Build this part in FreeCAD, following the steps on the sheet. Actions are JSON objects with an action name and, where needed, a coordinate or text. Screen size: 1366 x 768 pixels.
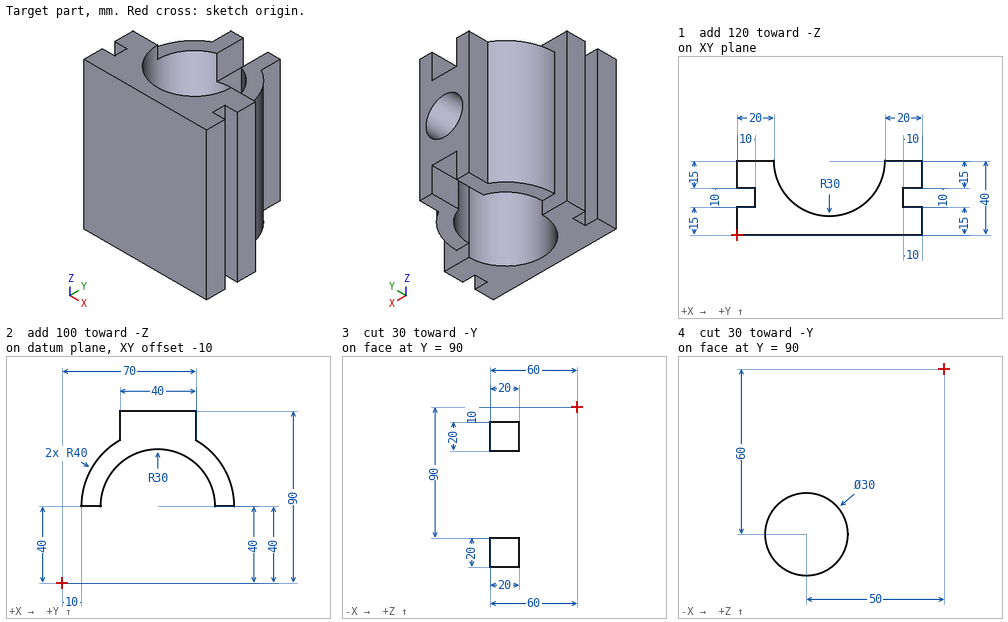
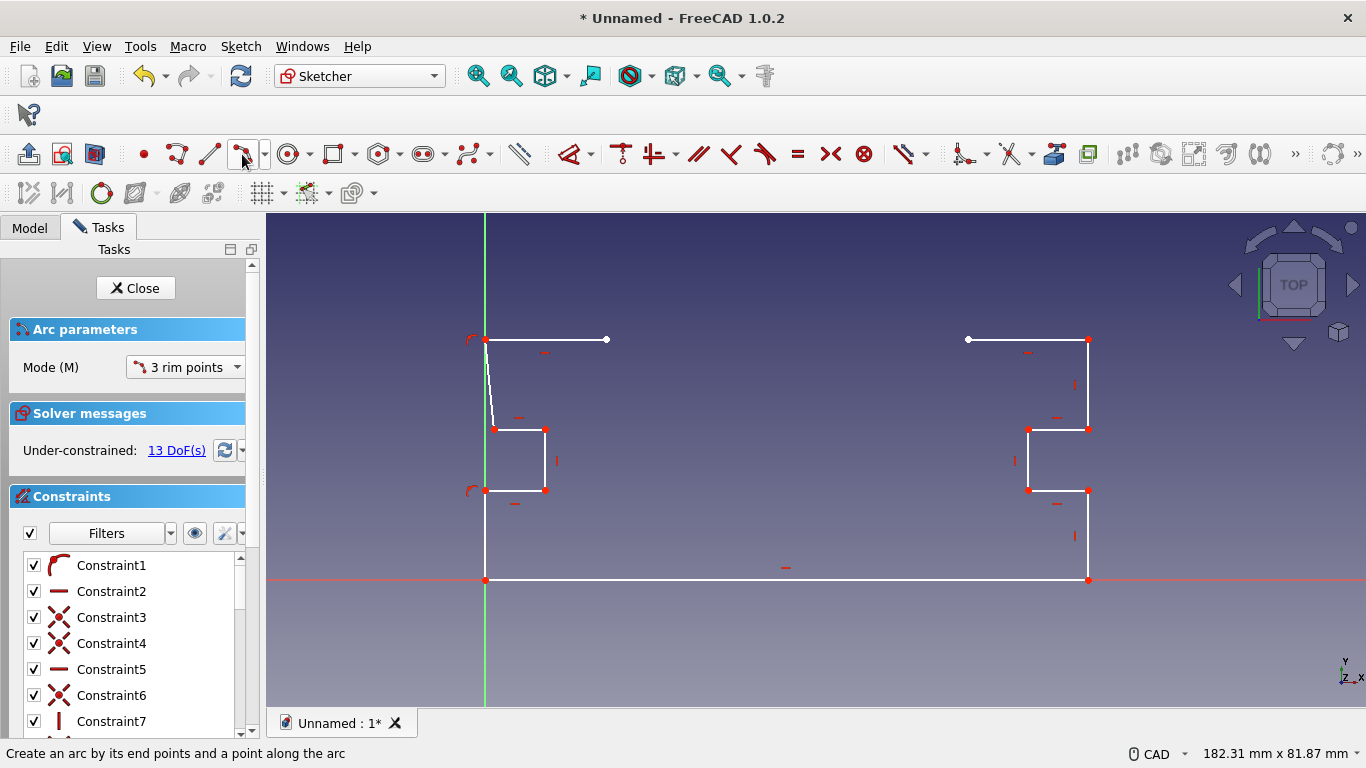
{"action": "left_click", "coordinate": [968, 340]}
{"action": "left_click", "coordinate": [606, 340]}
{"action": "left_click", "coordinate": [787, 520]}
{"action": "key", "text": "Escape"}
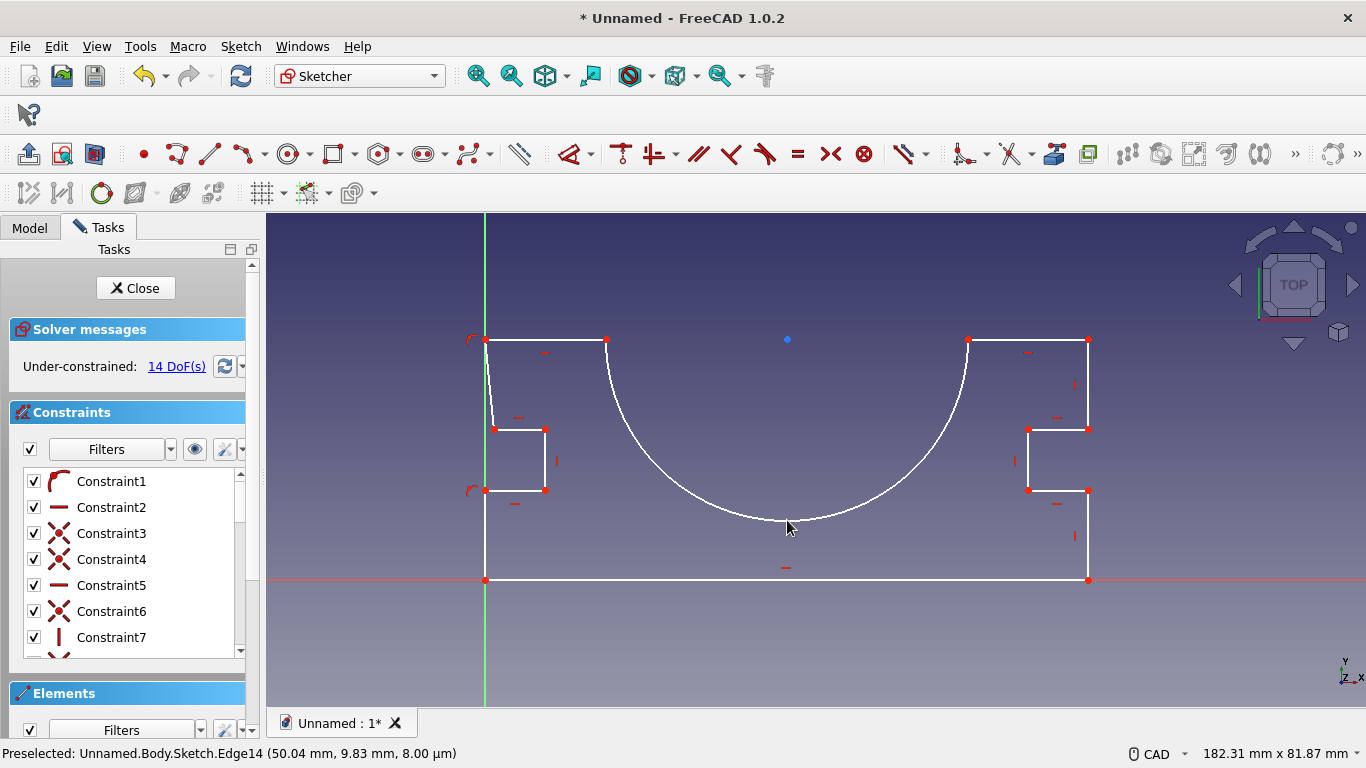
{"action": "left_click", "coordinate": [488, 367]}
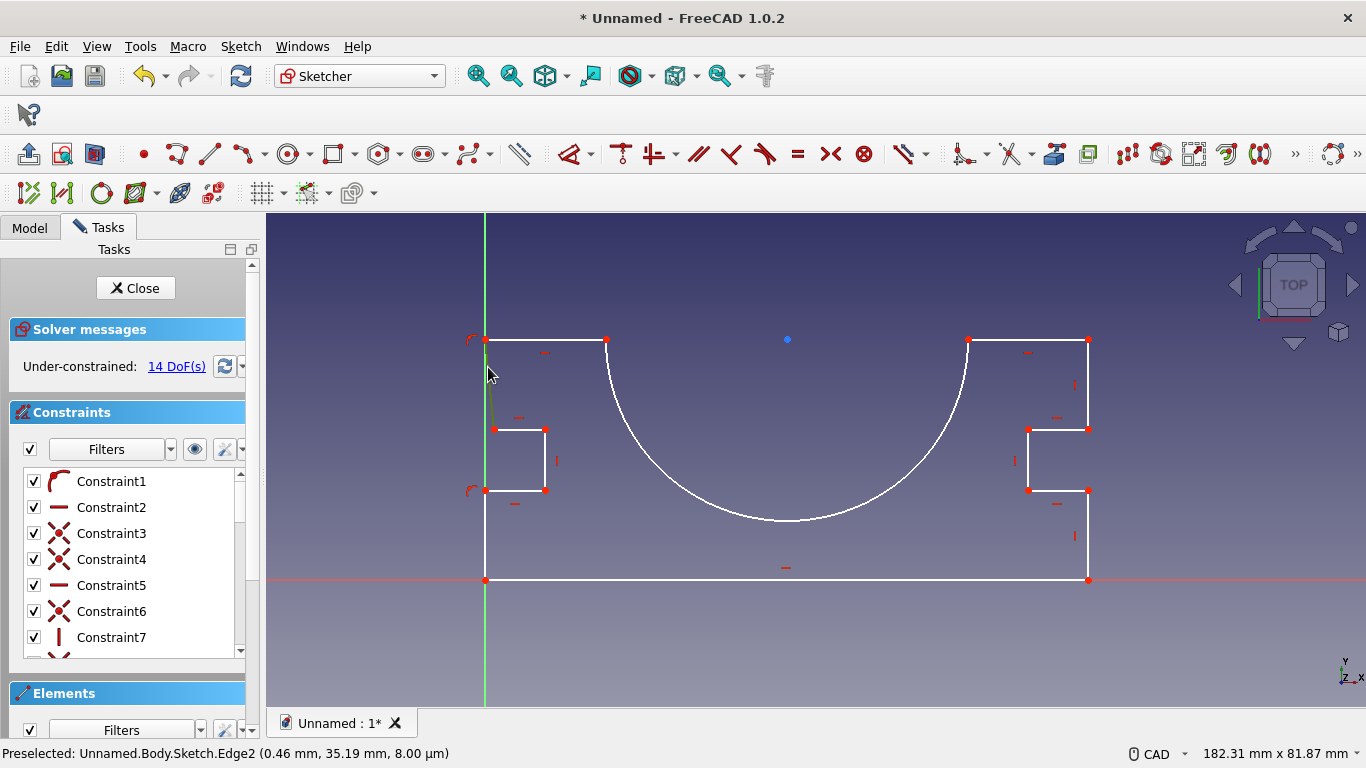
{"action": "left_click", "coordinate": [676, 154]}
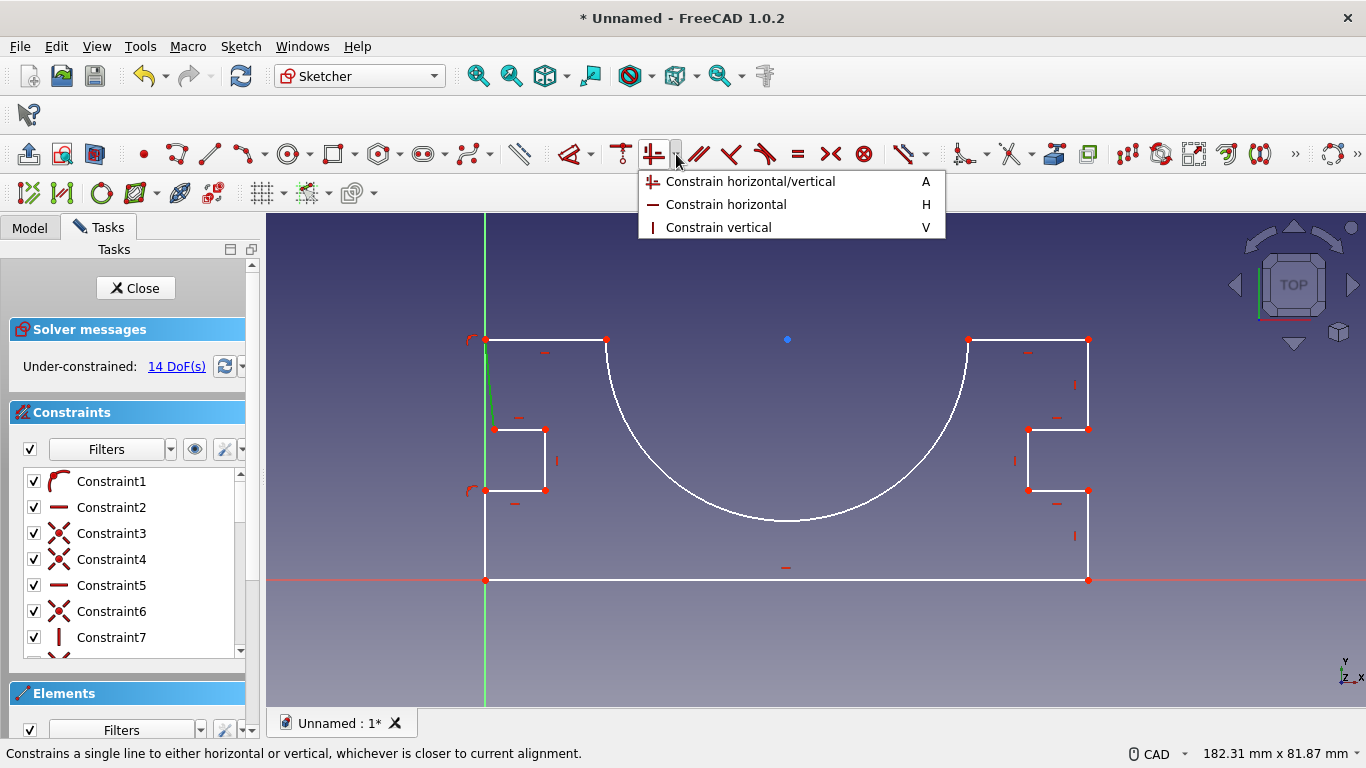
{"action": "left_click", "coordinate": [792, 228]}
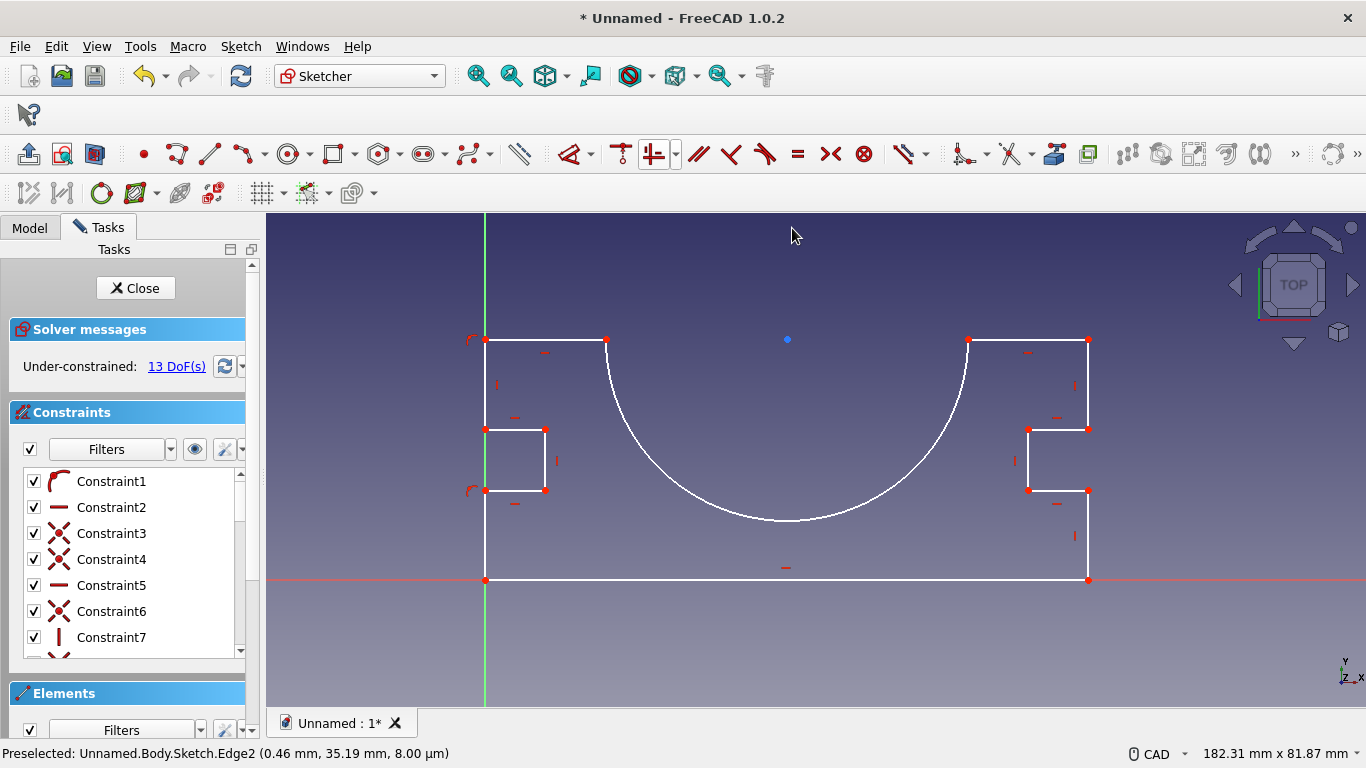
{"action": "left_click", "coordinate": [568, 154]}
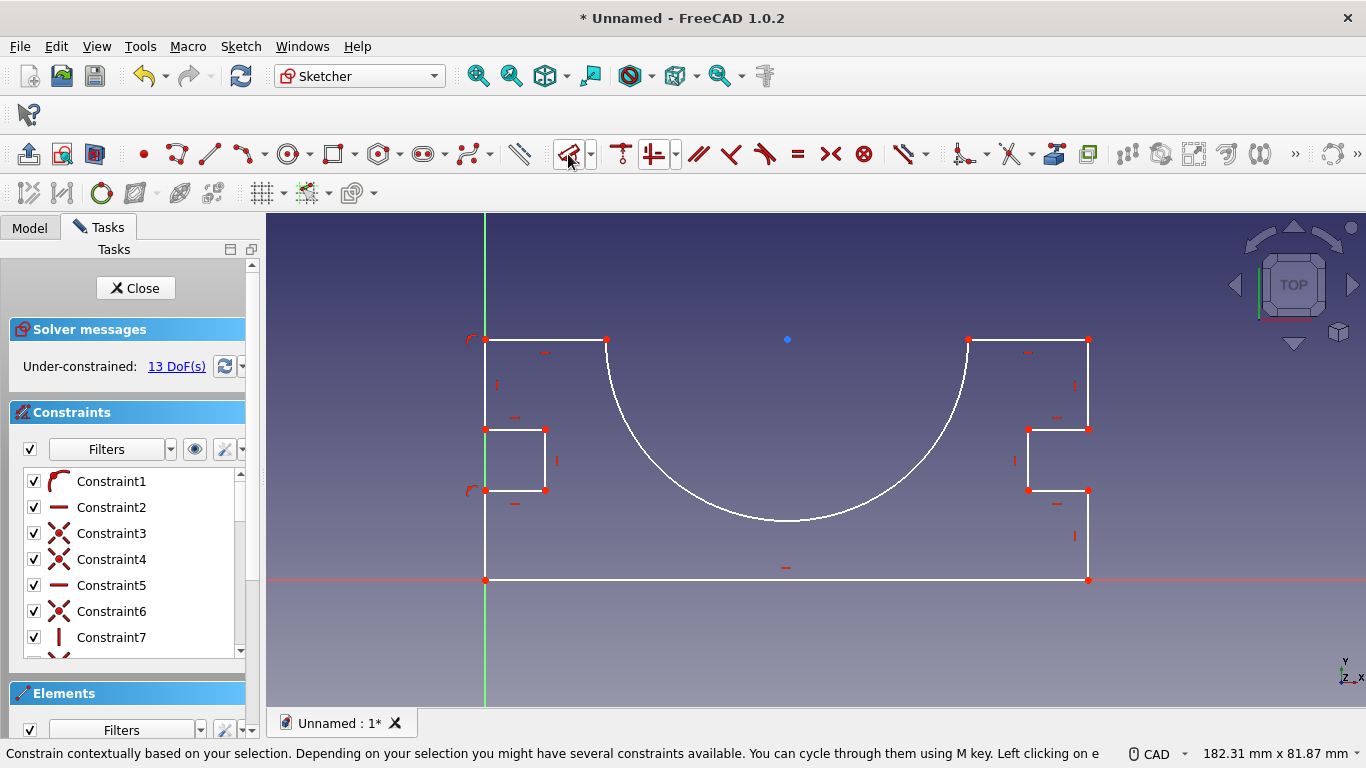
{"action": "left_click", "coordinate": [681, 486]}
{"action": "left_click", "coordinate": [662, 512]}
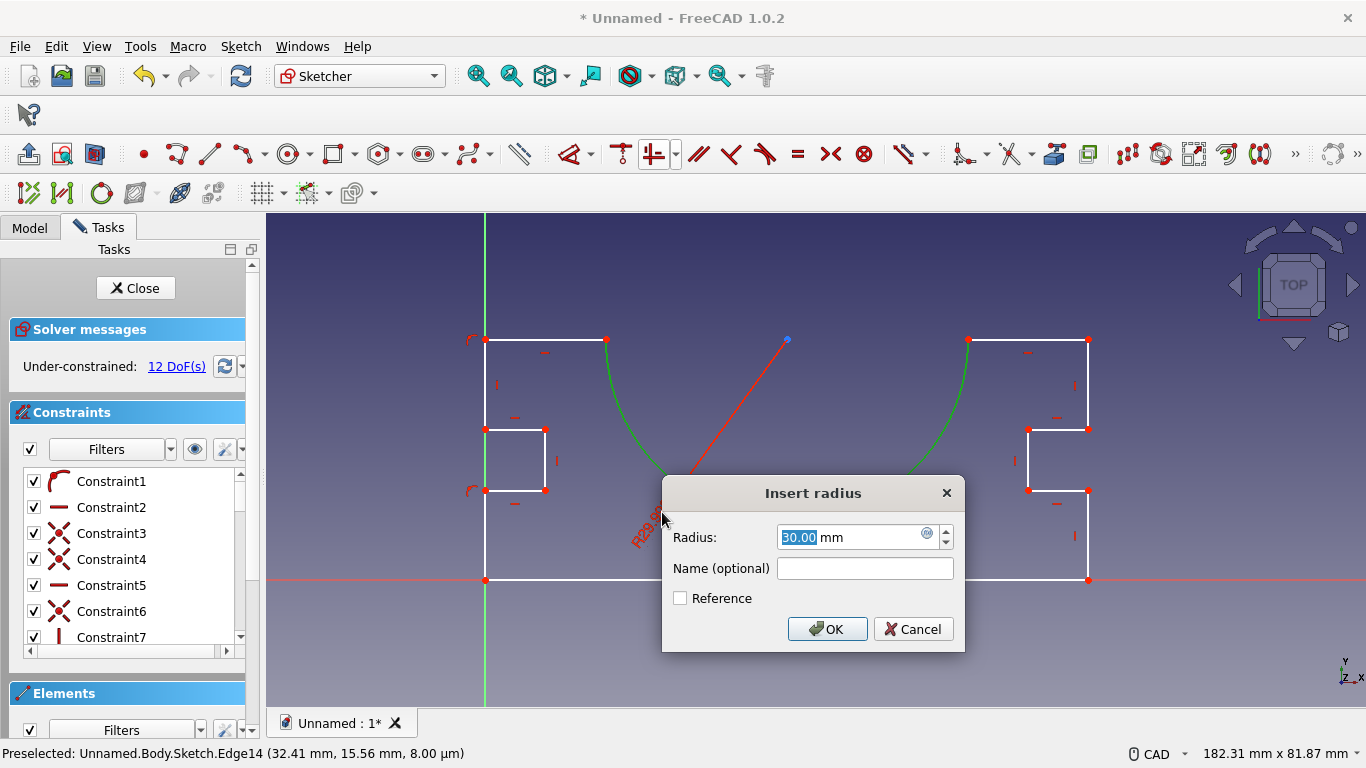
{"action": "type", "text": "30"}
{"action": "key", "text": "Return"}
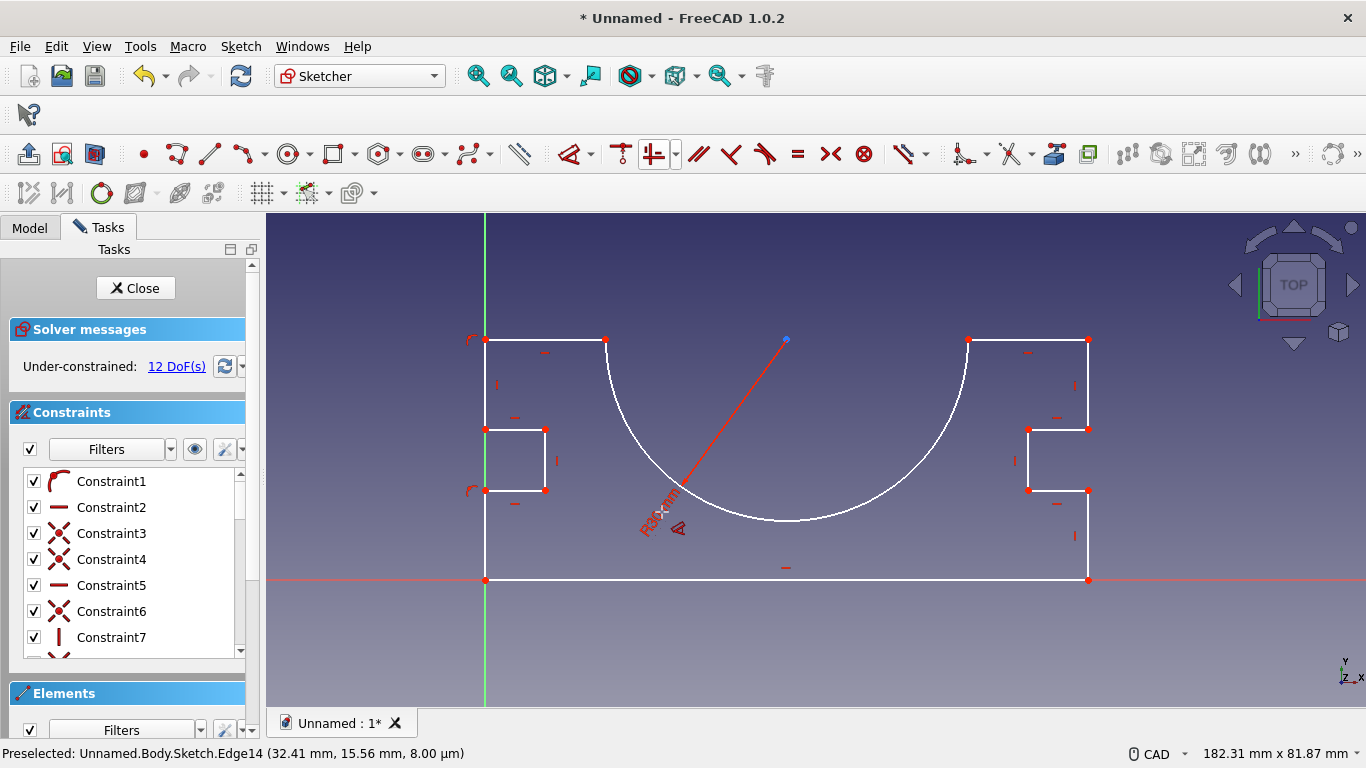
{"action": "left_click", "coordinate": [570, 340]}
{"action": "left_click", "coordinate": [546, 306]}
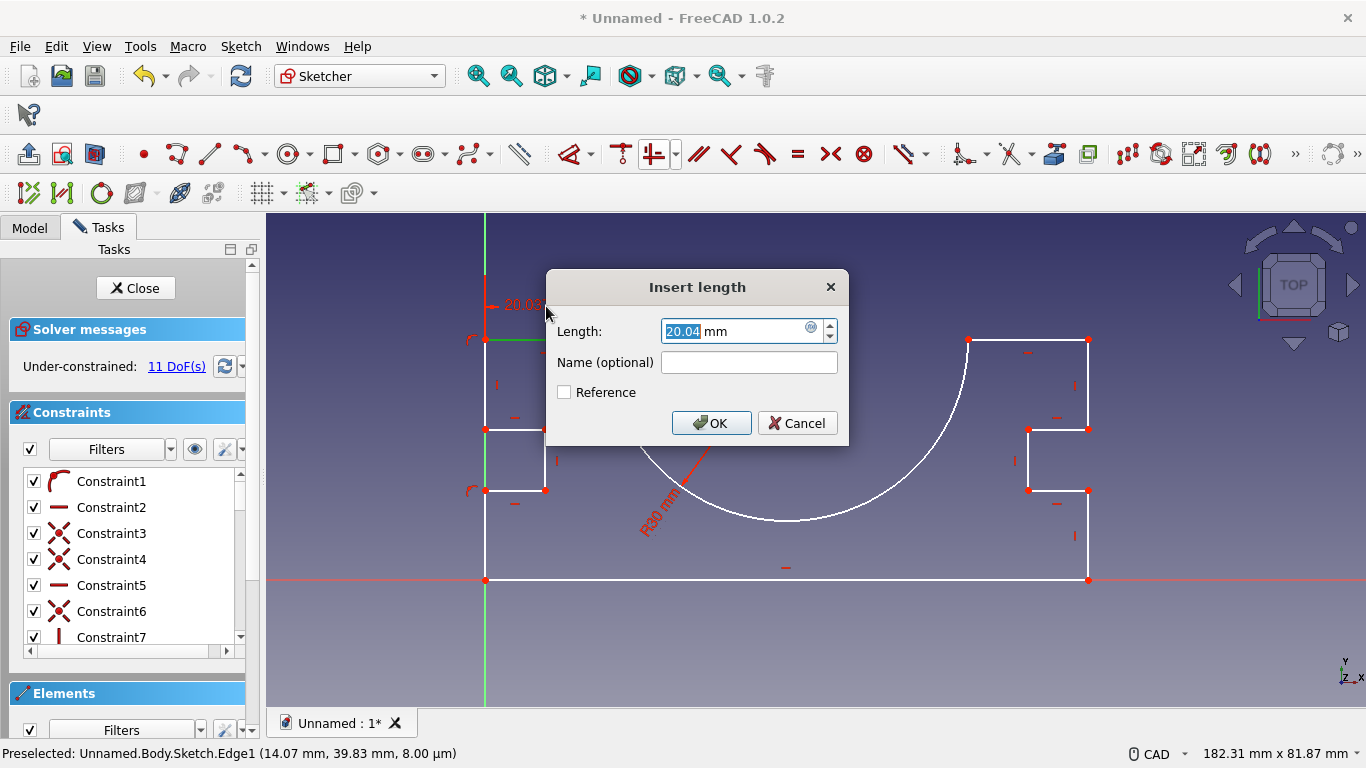
{"action": "type", "text": "20"}
{"action": "key", "text": "Return"}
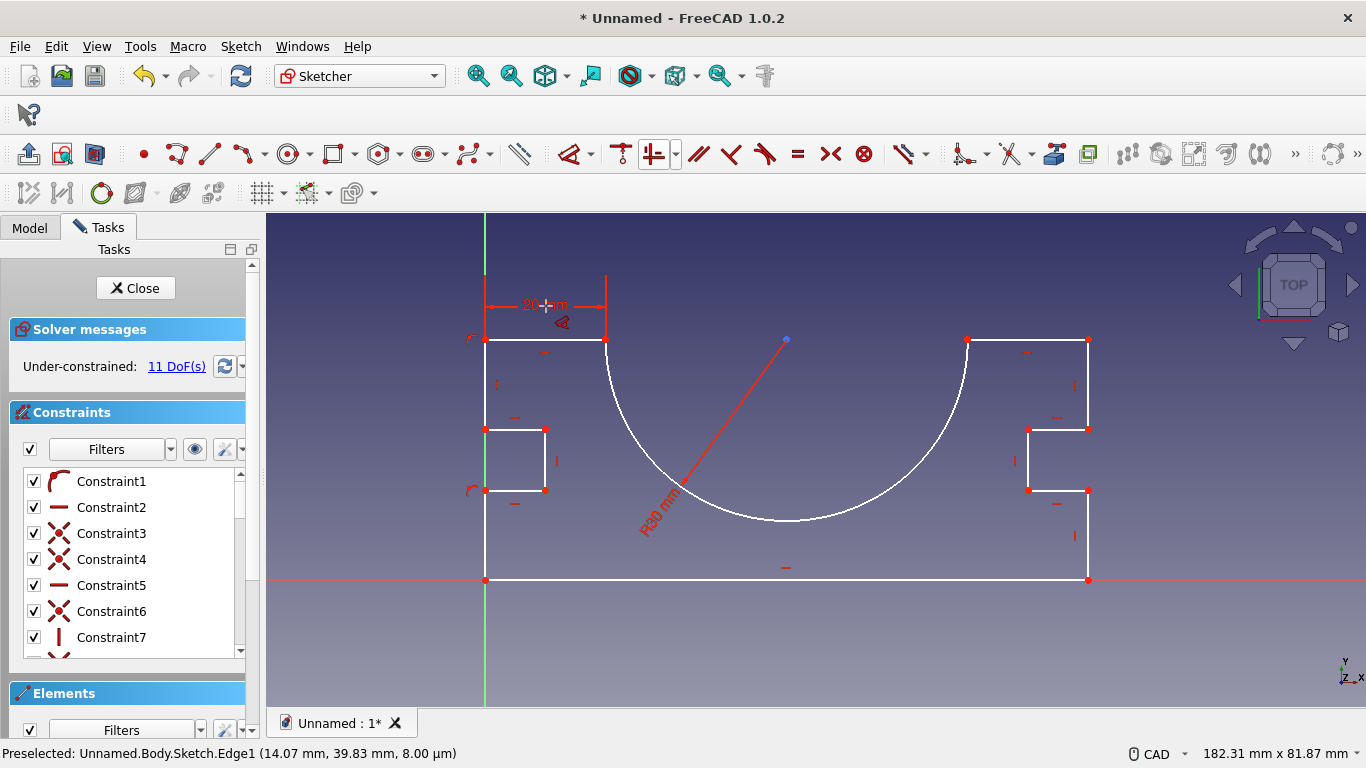
{"action": "left_click", "coordinate": [485, 367]}
{"action": "left_click", "coordinate": [451, 385]}